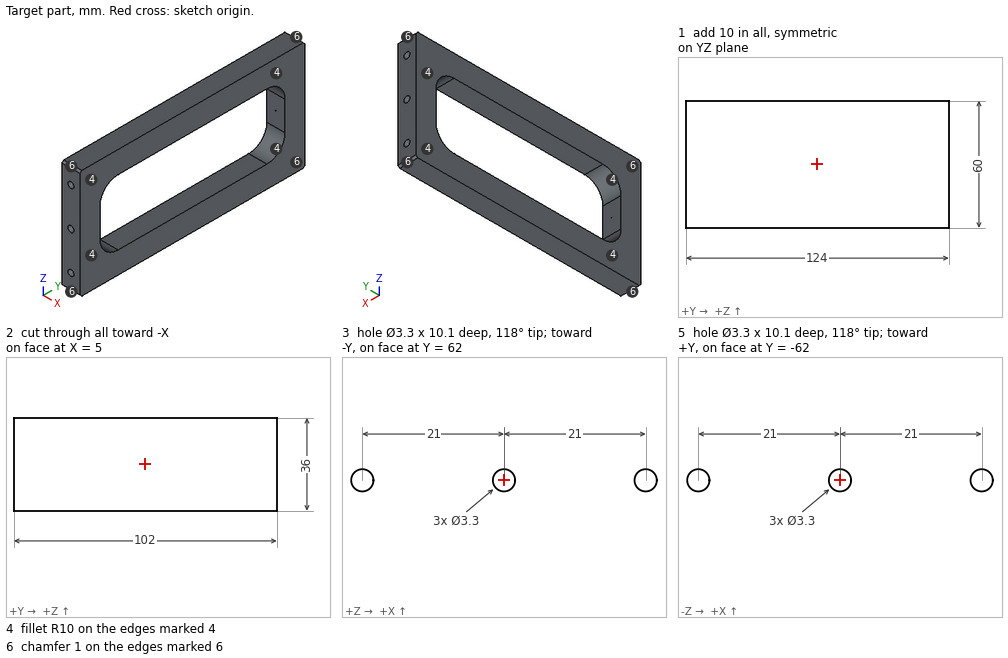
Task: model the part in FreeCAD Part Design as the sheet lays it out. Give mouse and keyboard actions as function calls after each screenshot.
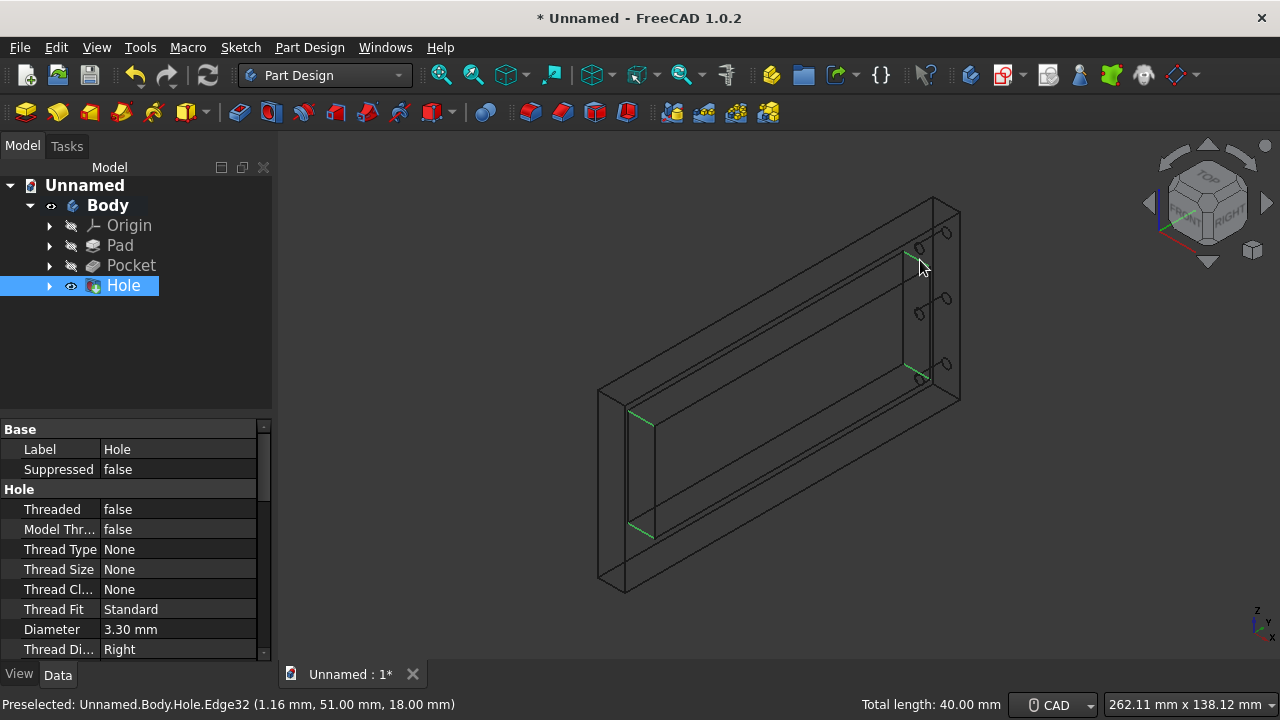
key(v)
key(1)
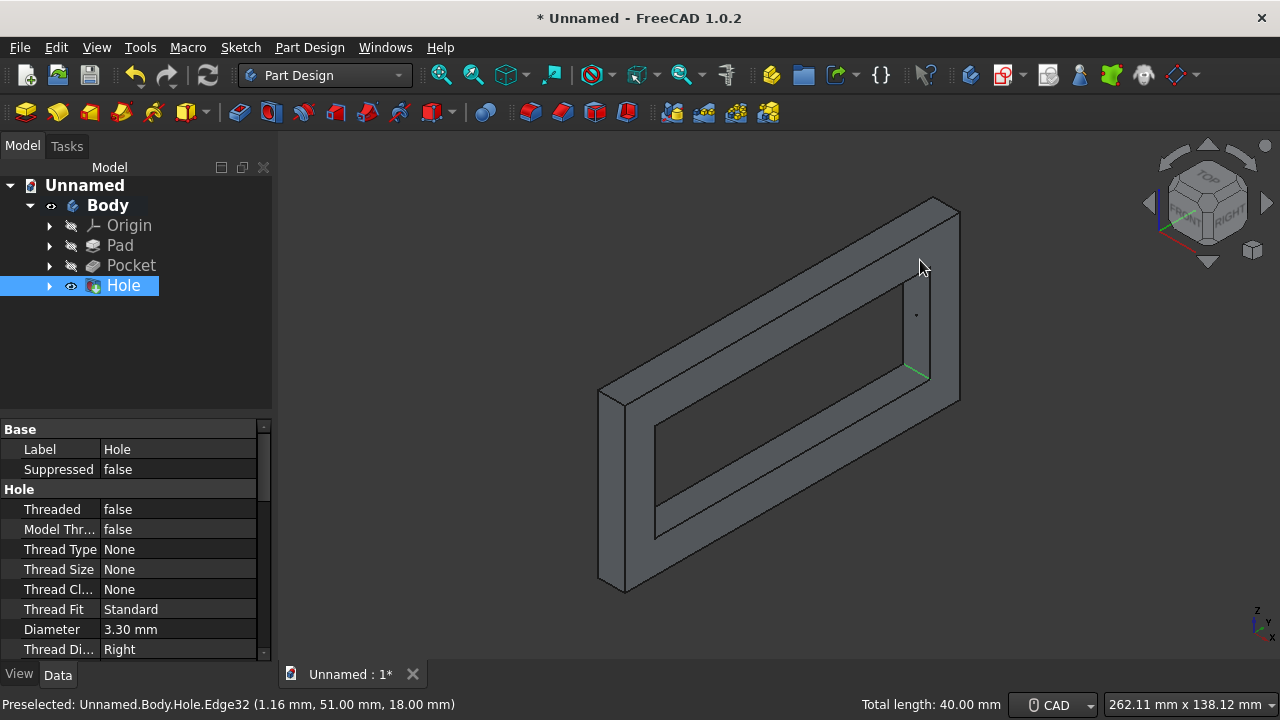
click(532, 112)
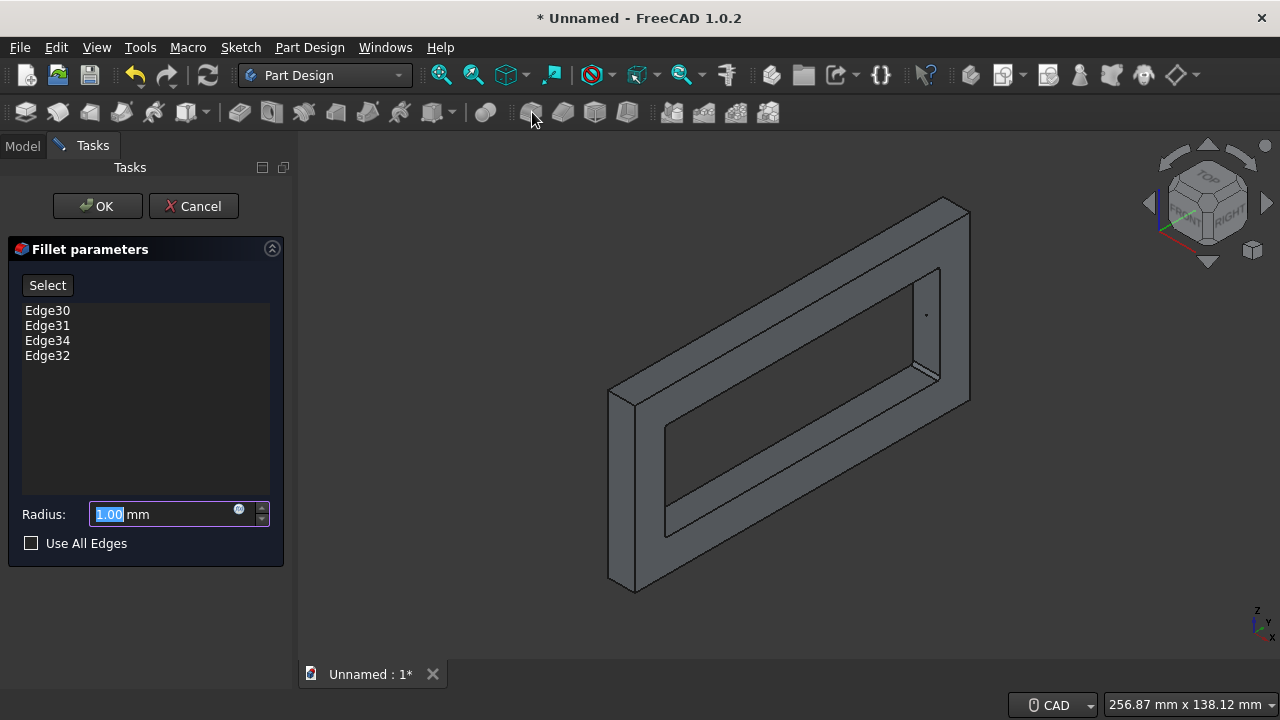
text(10)
key(Tab)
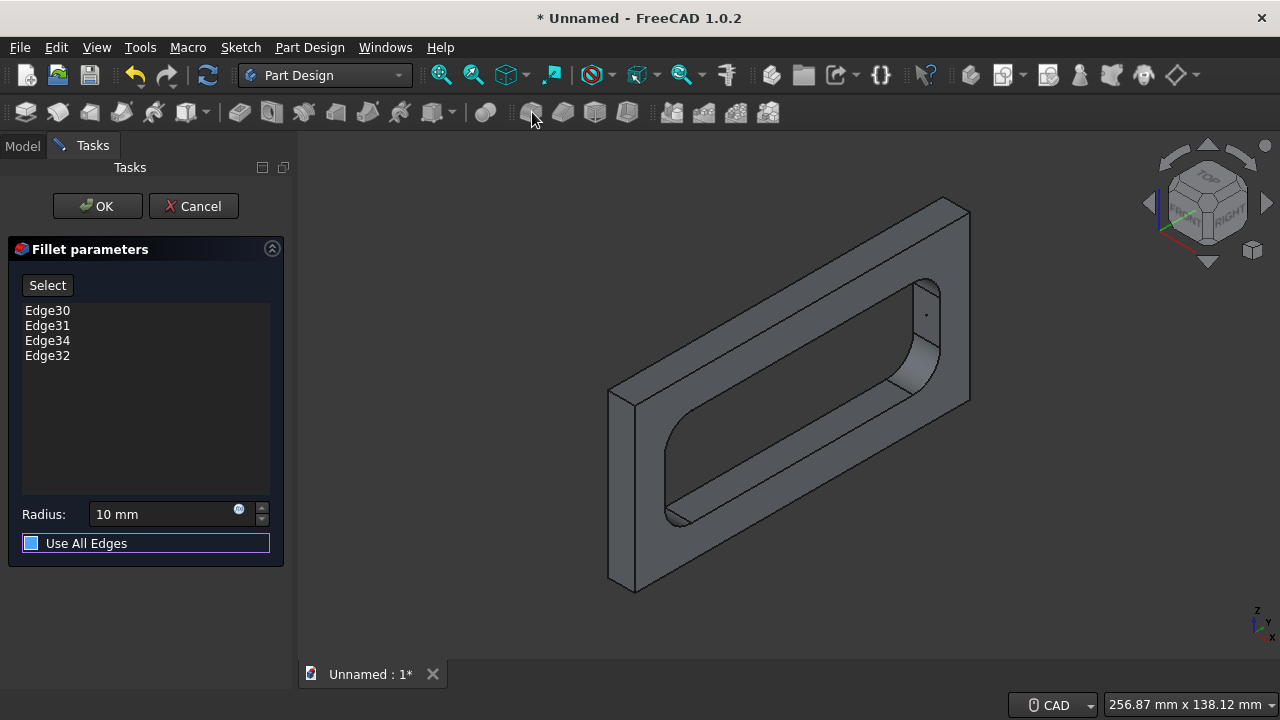
click(98, 206)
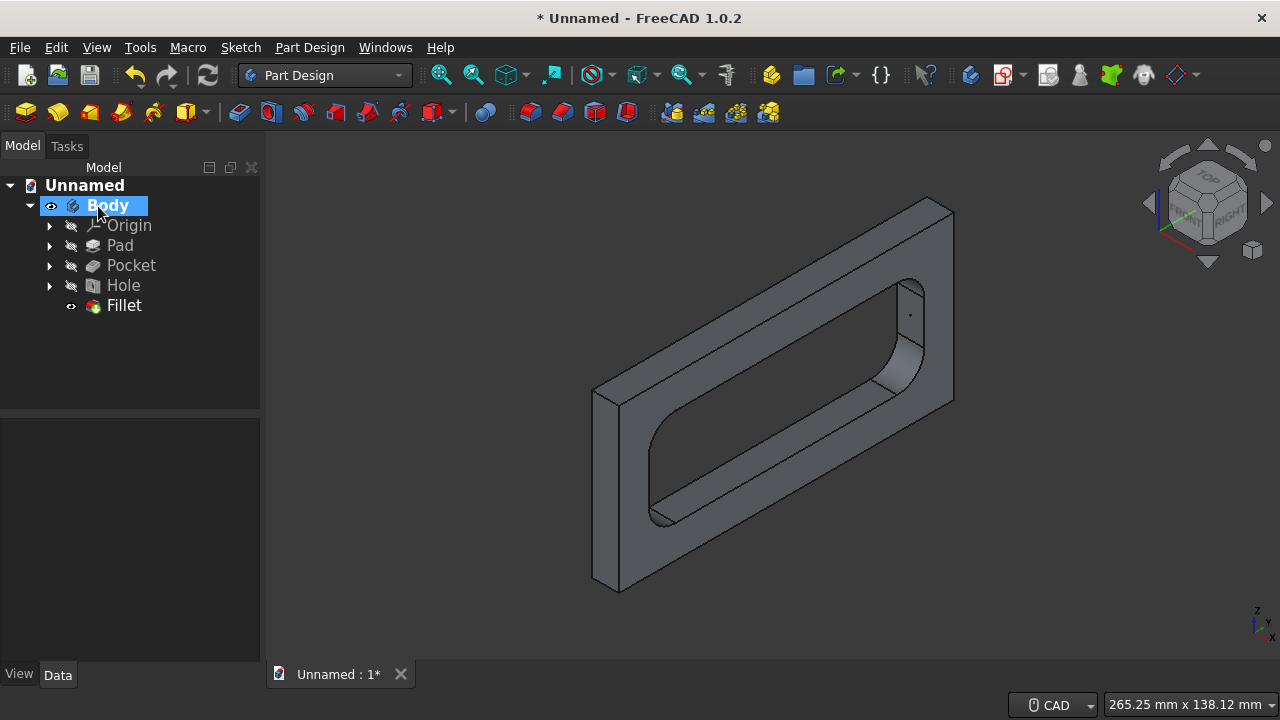
click(605, 544)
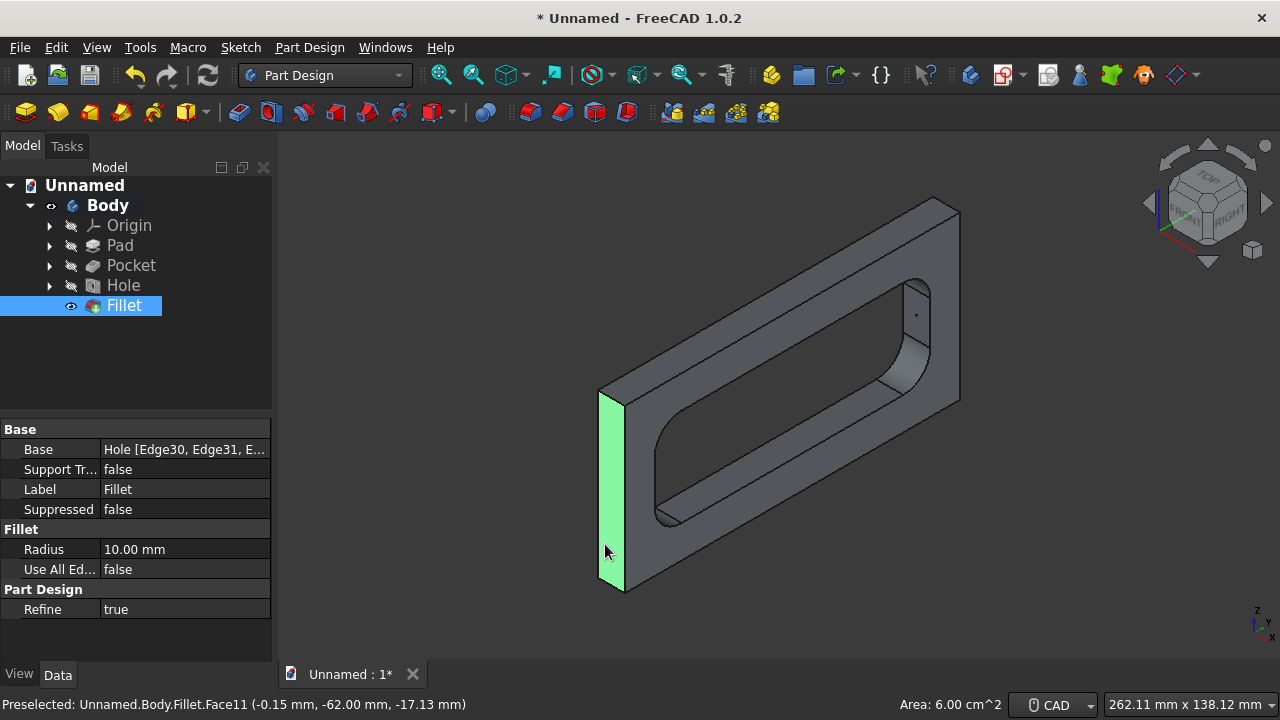
click(1004, 76)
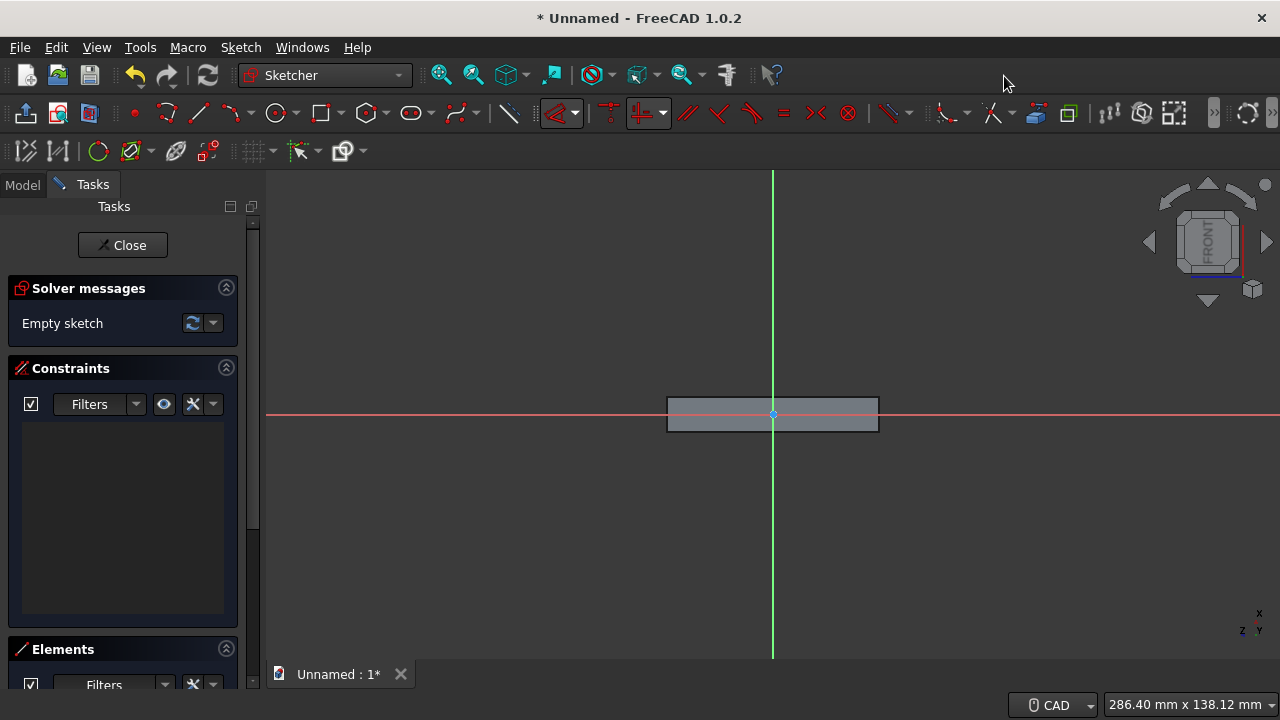
scroll(803, 415, up, 6)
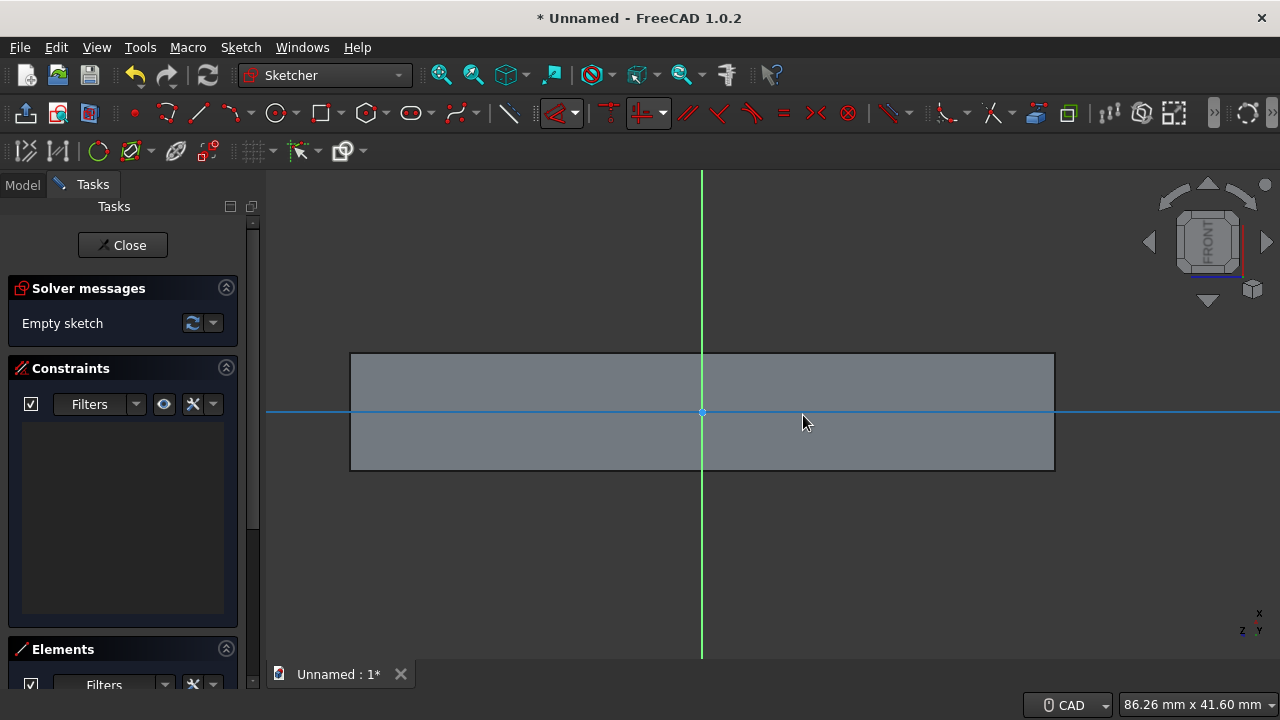
key(g)
key(c)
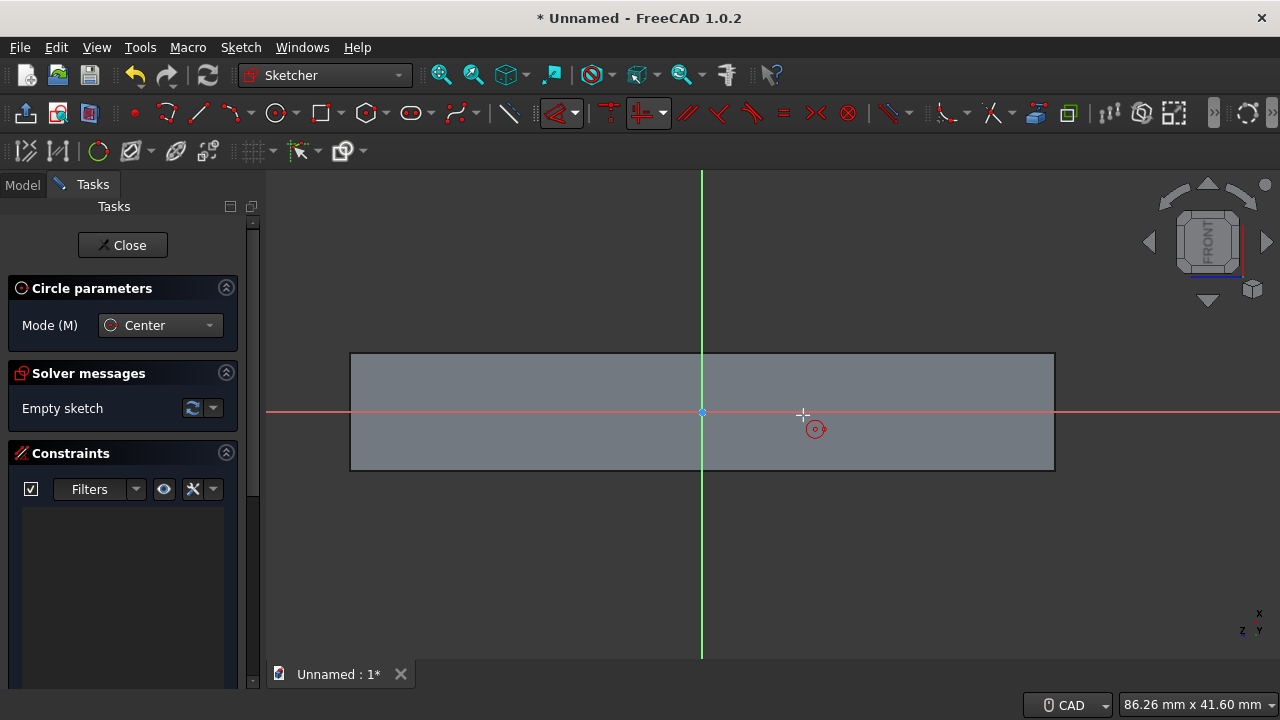
click(702, 412)
move(716, 398)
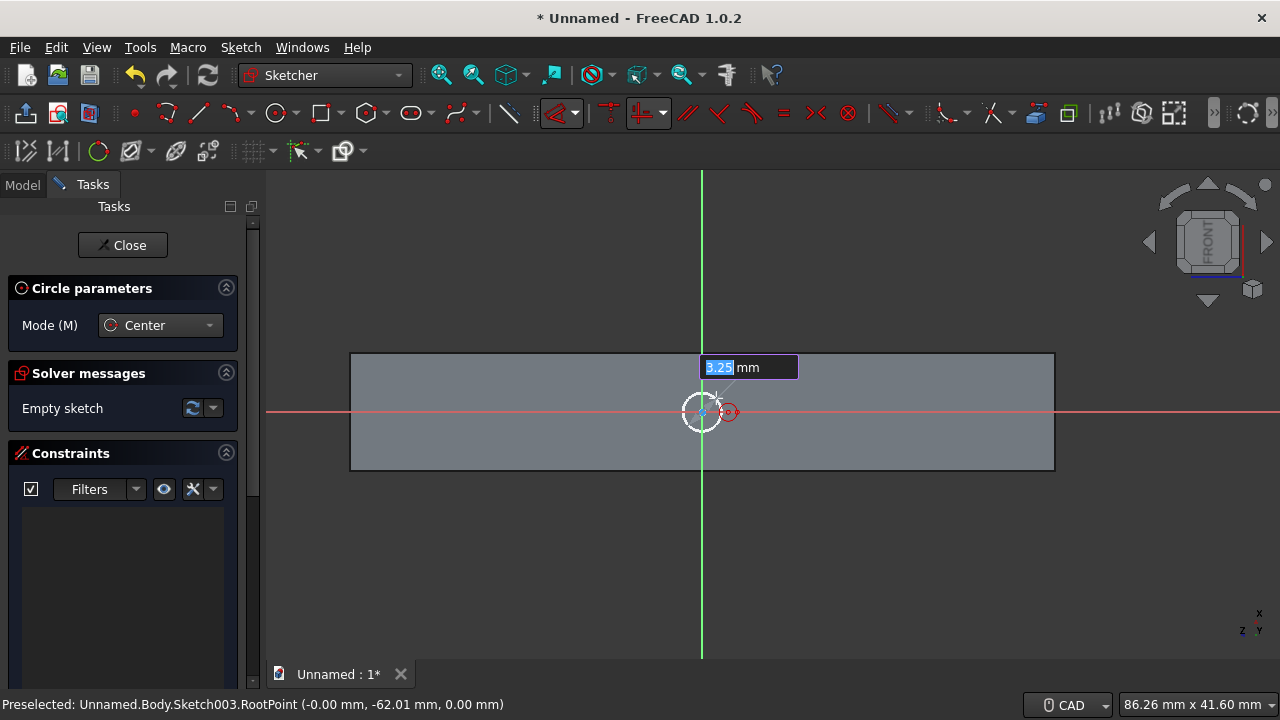
text(3.3)
key(Return)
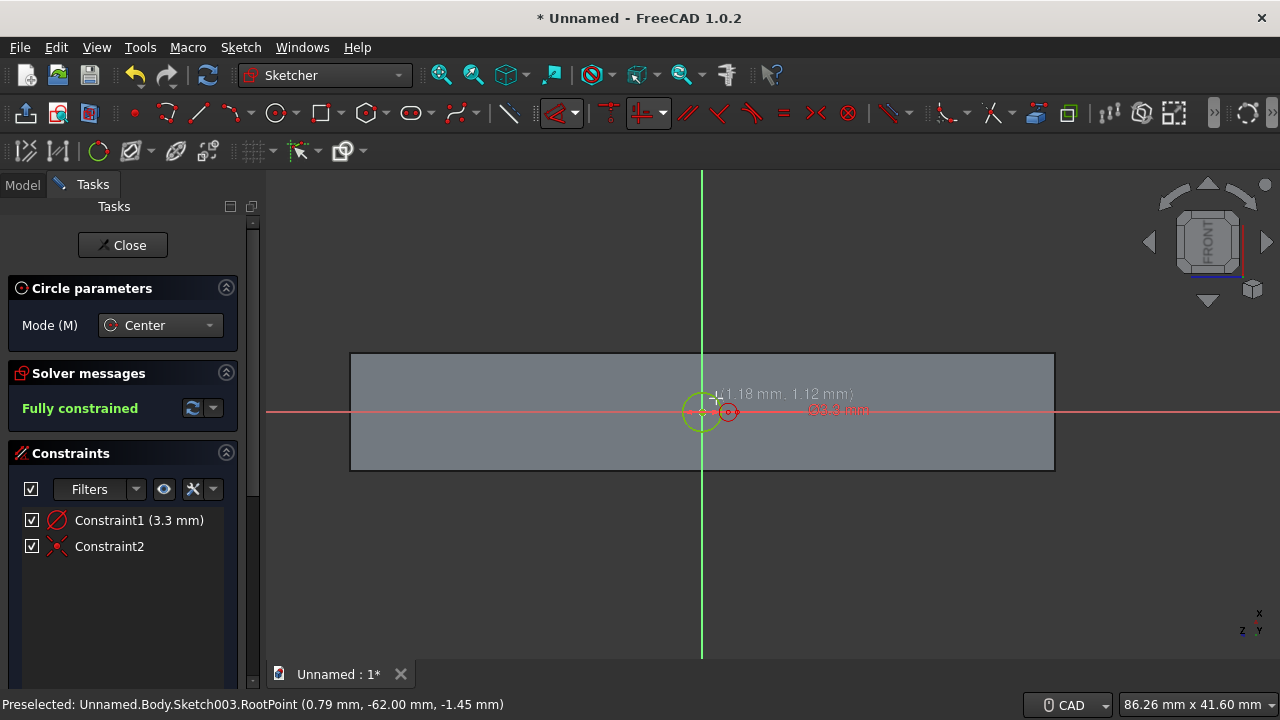
click(949, 412)
move(956, 394)